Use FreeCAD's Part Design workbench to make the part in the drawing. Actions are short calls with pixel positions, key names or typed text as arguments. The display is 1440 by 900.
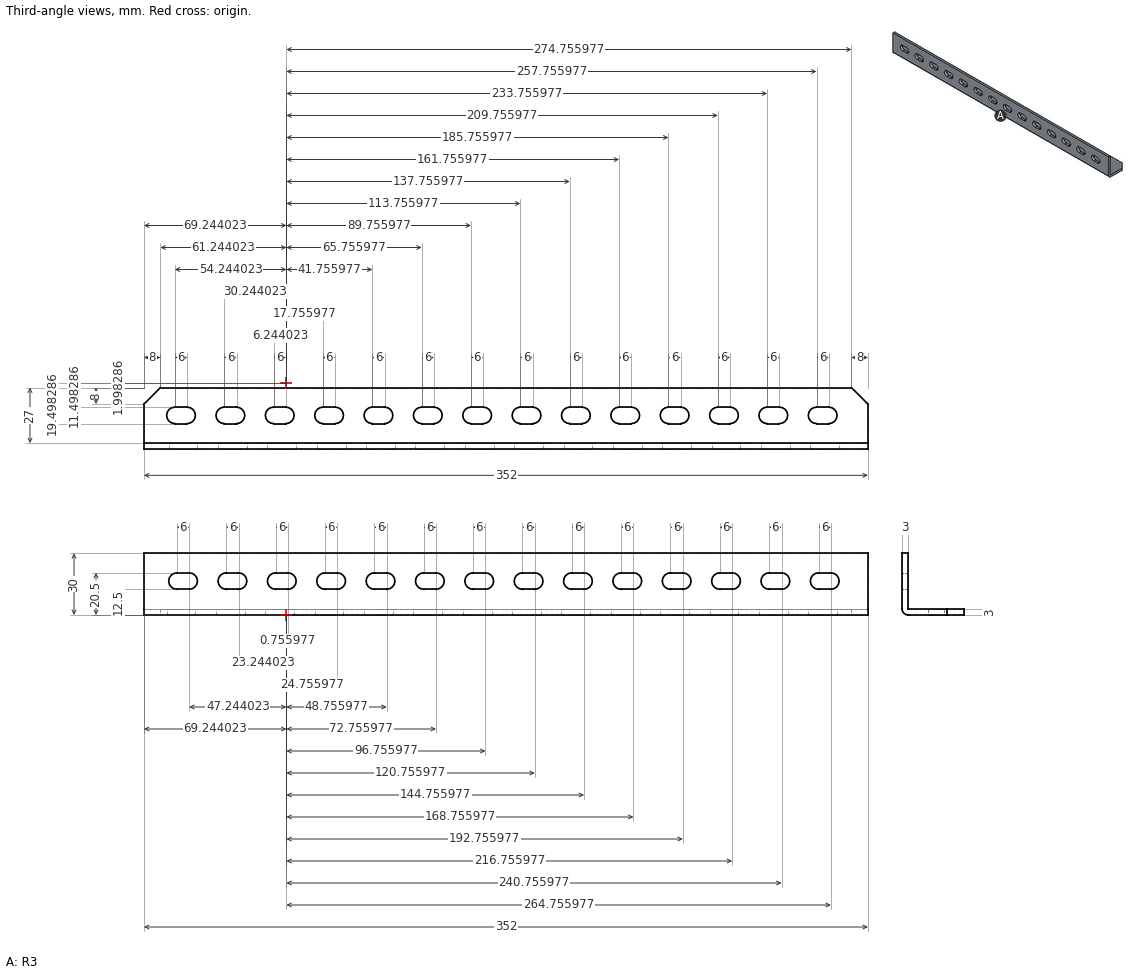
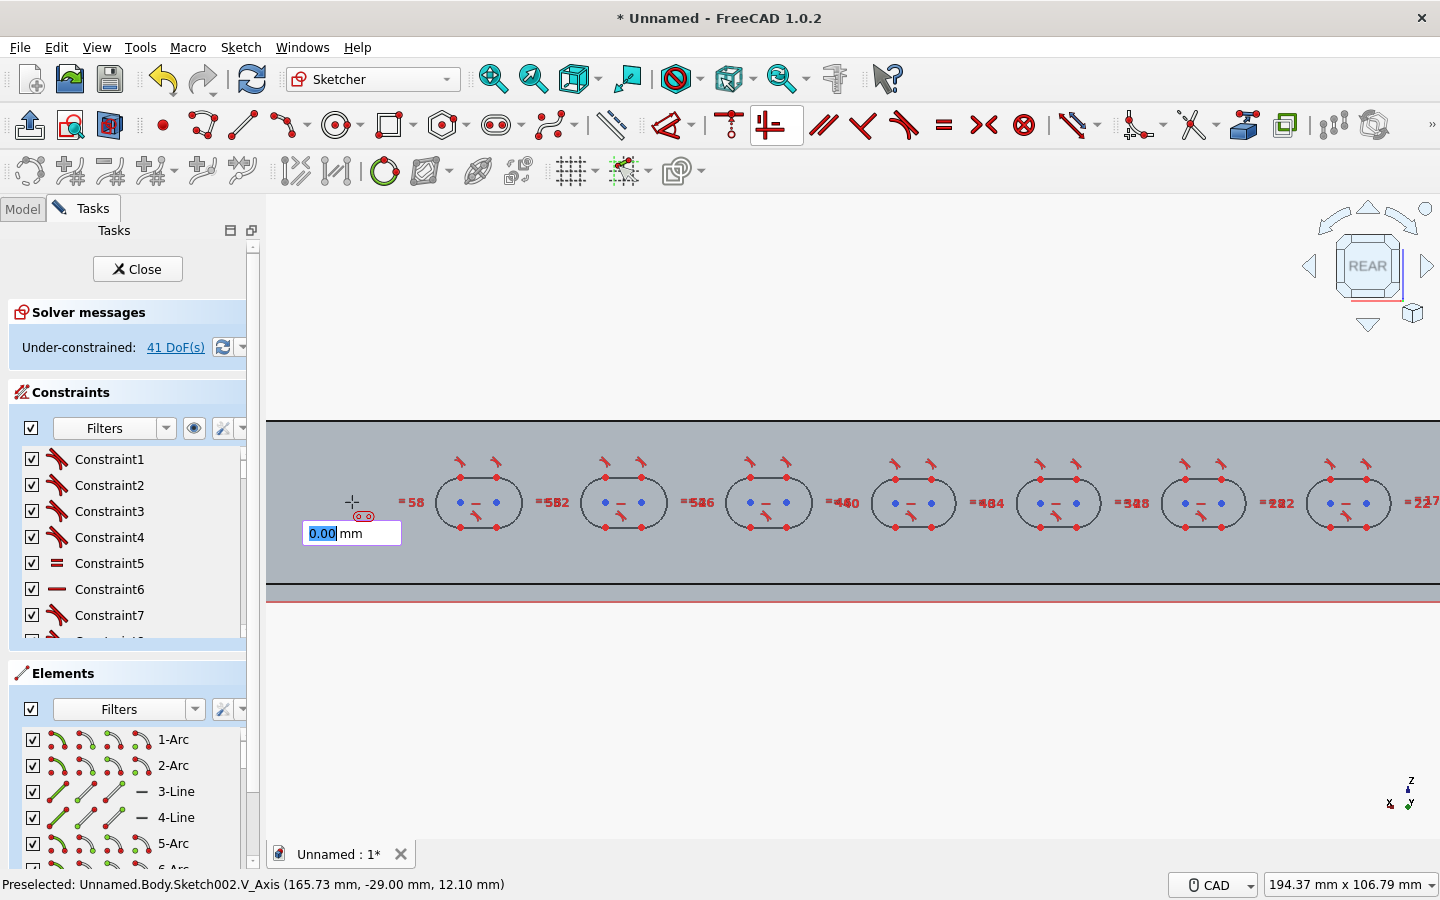
click(334, 527)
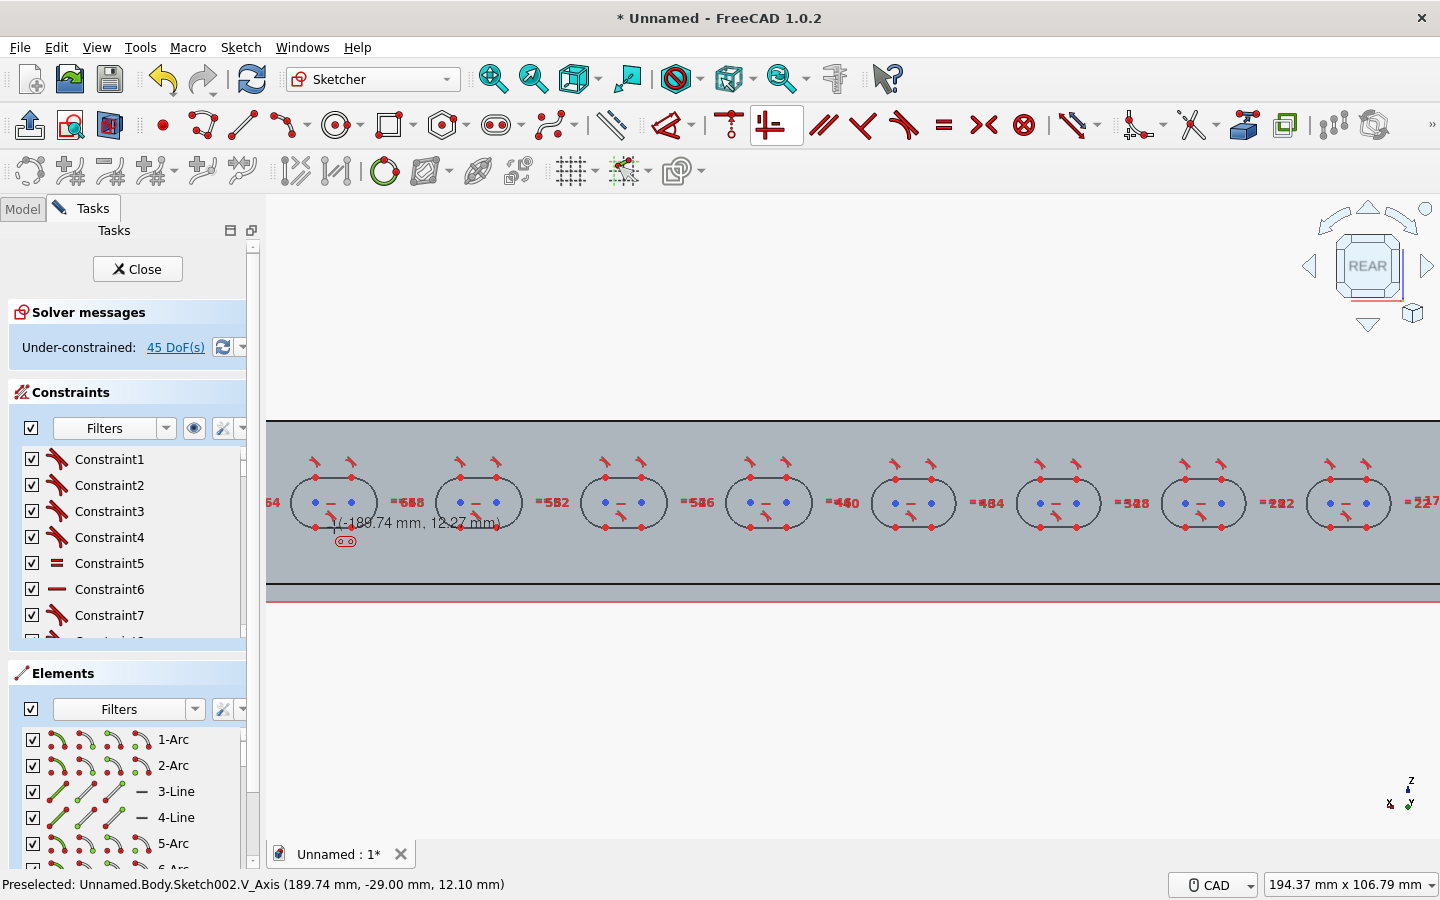
scroll(751, 503, down, 5)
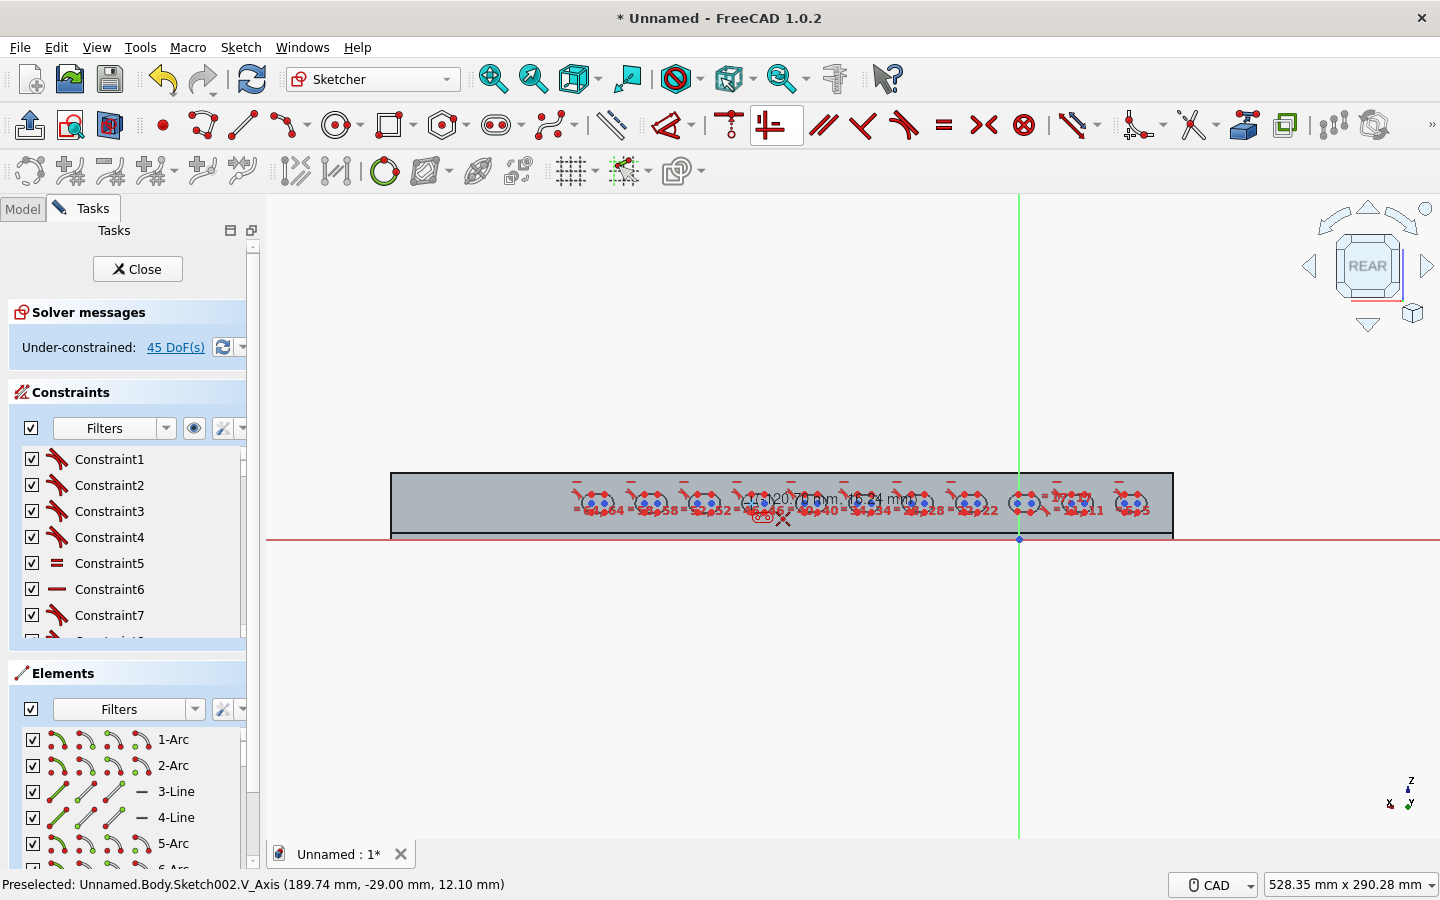
scroll(538, 503, up, 5)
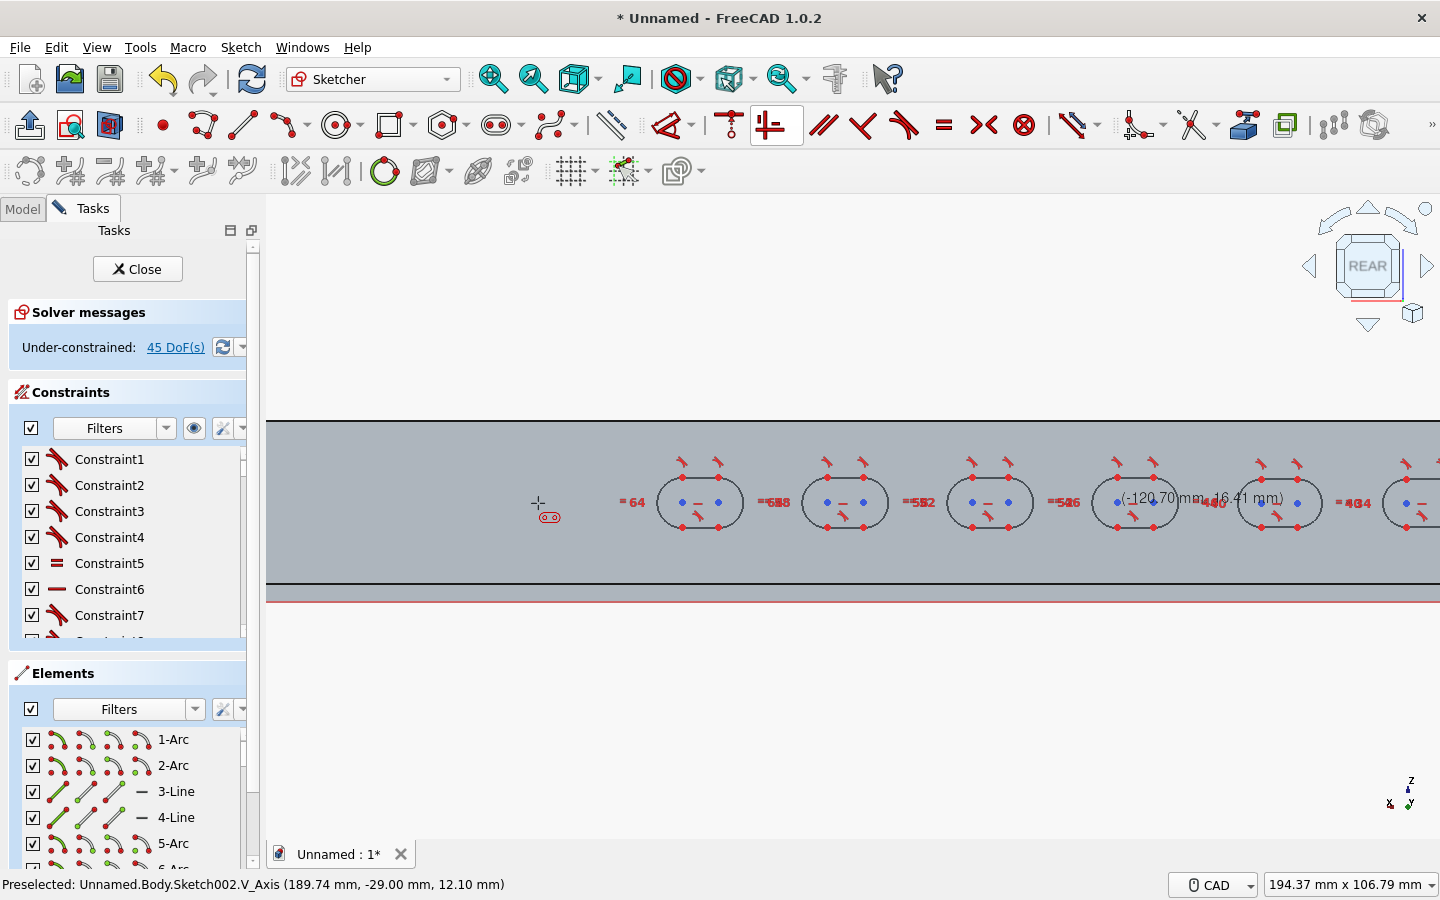
click(537, 502)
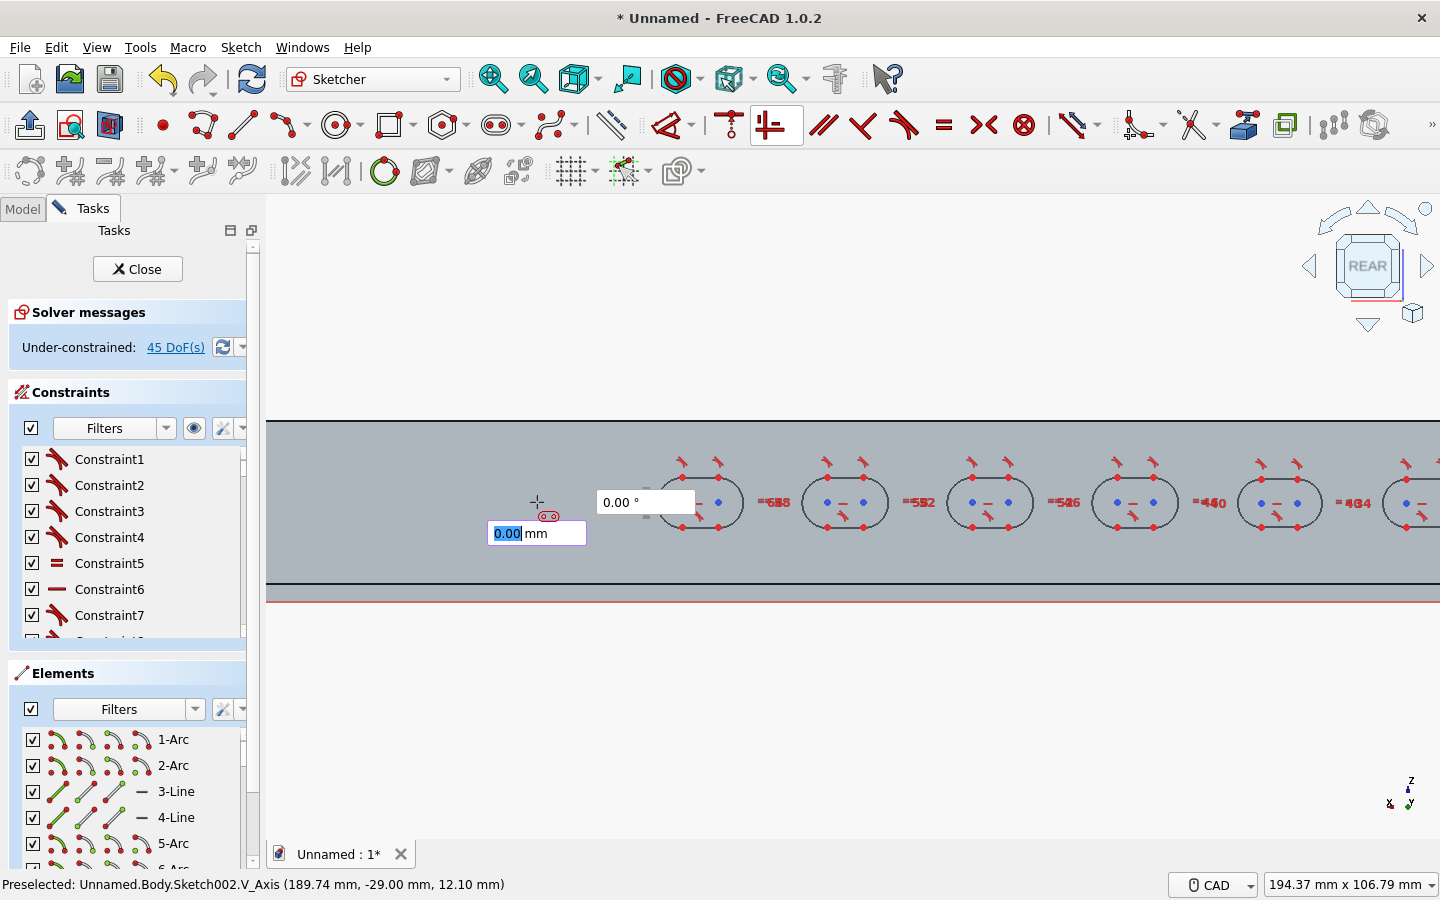
click(573, 502)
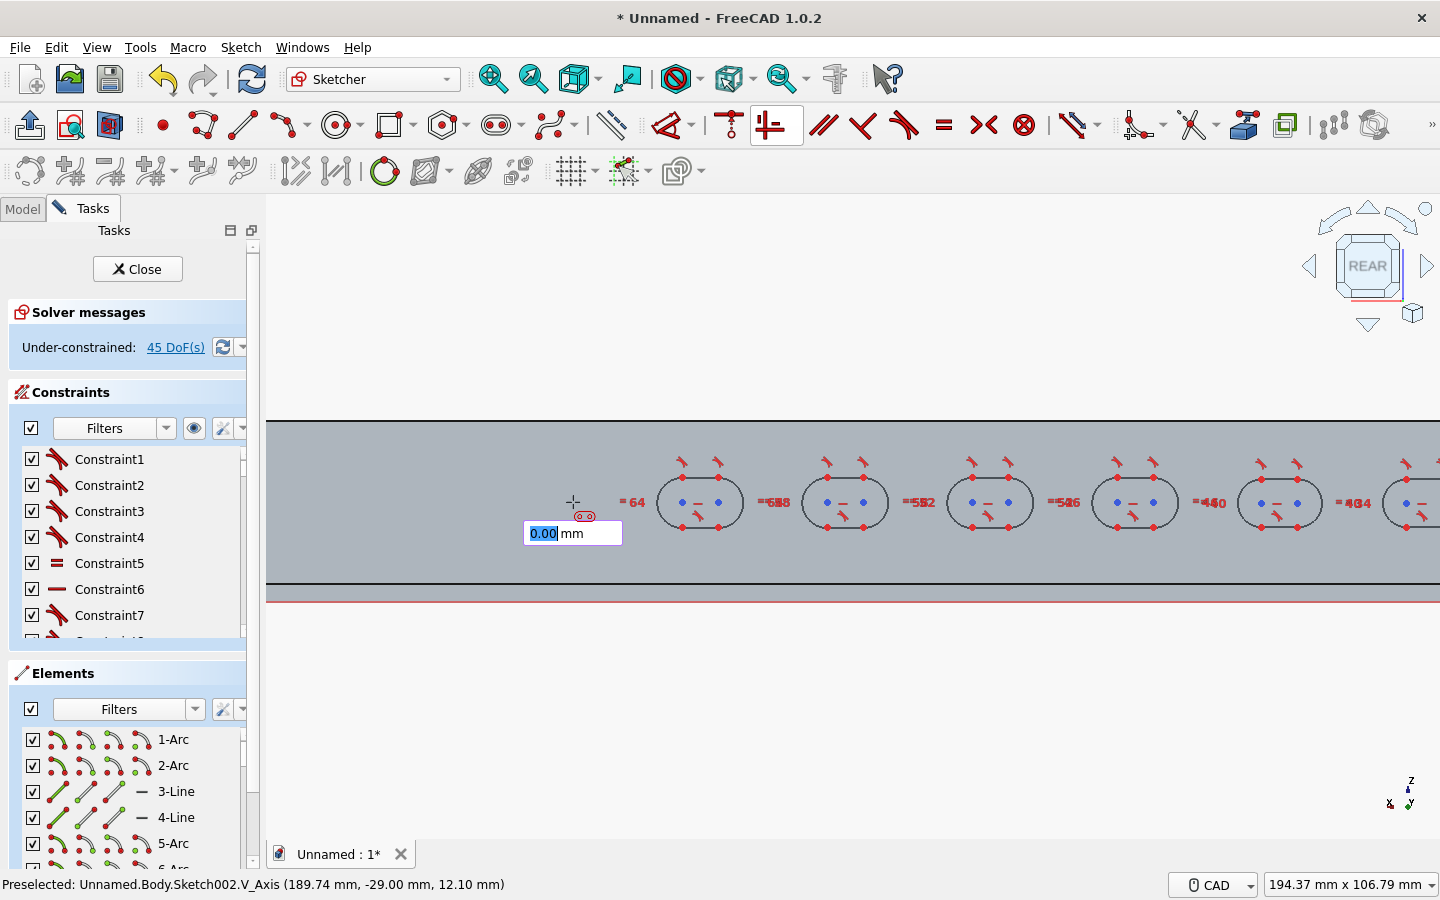
click(555, 527)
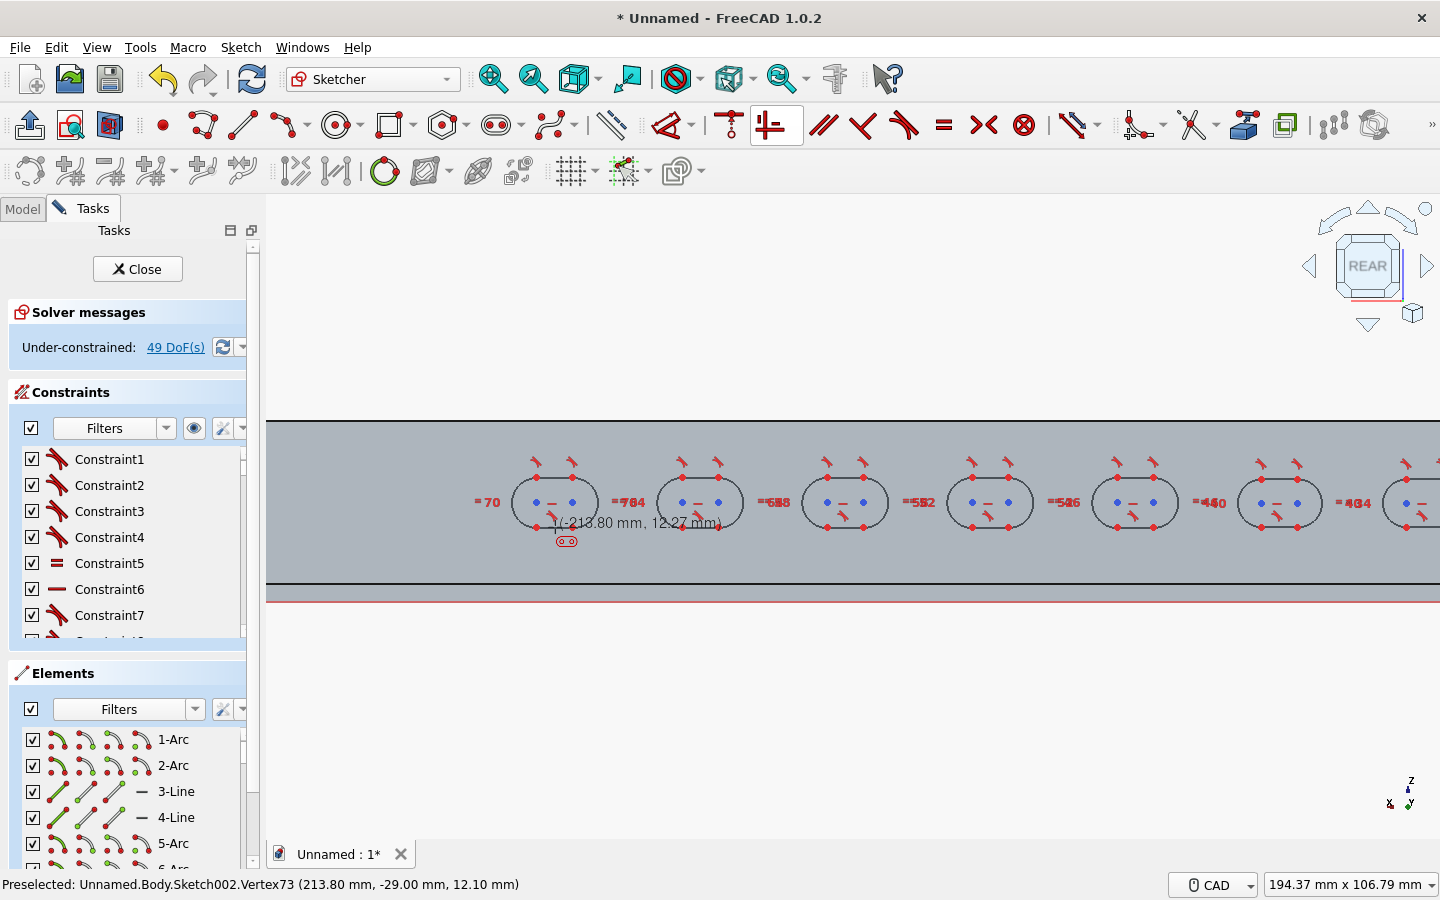
click(392, 502)